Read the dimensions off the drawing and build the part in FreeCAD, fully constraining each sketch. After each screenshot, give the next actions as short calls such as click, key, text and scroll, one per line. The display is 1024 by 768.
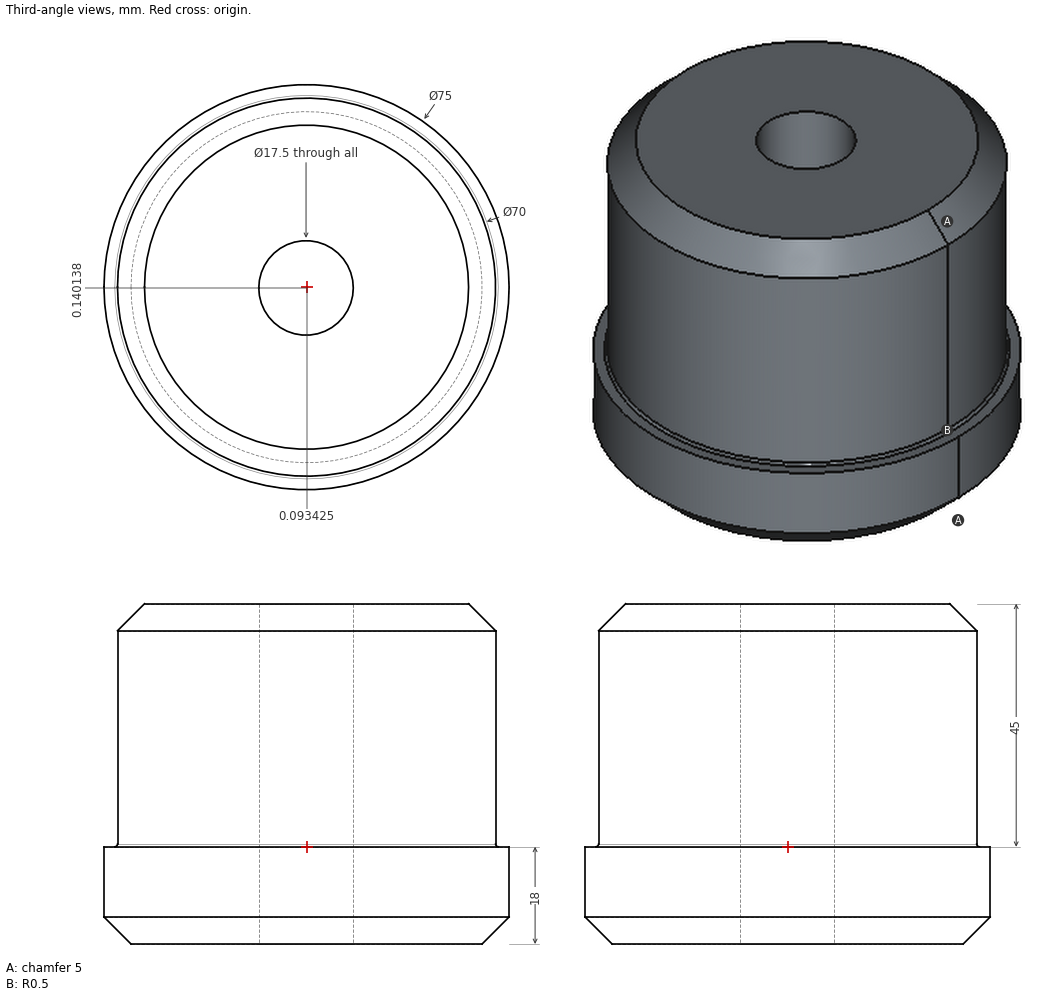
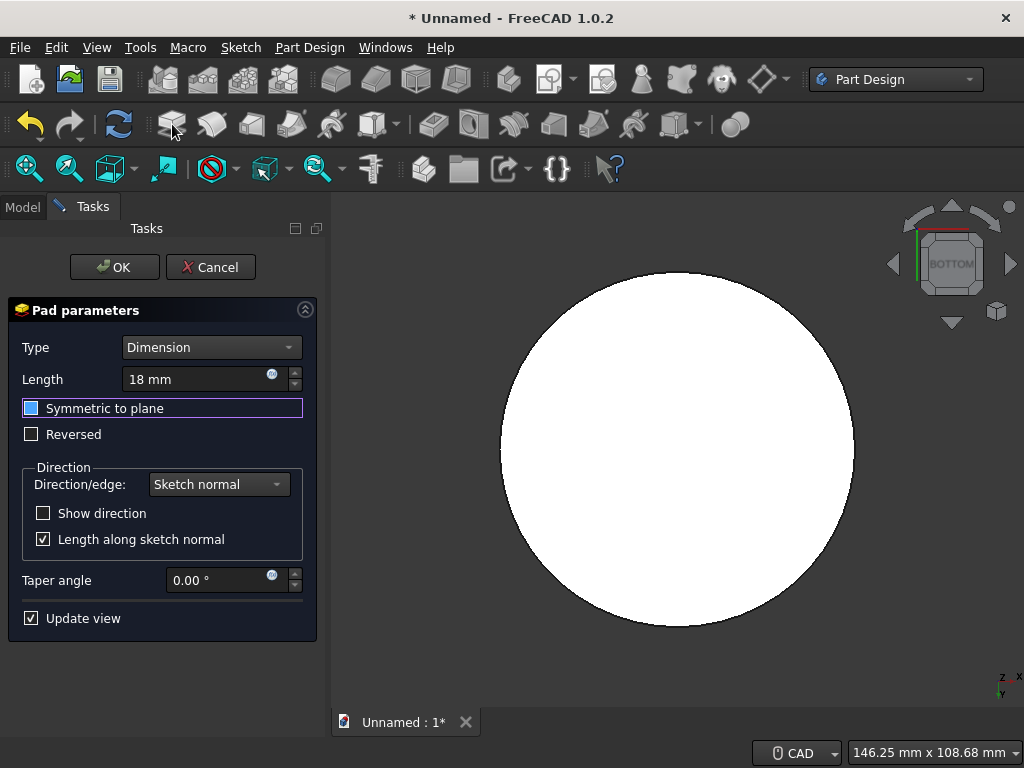
click(115, 267)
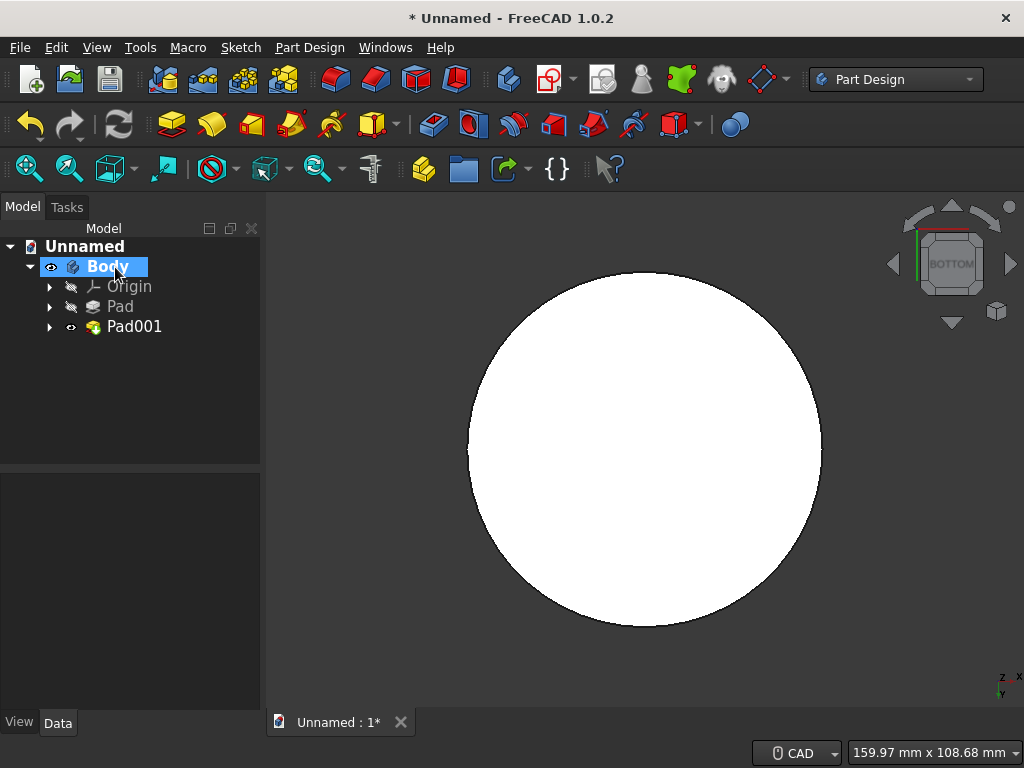
click(467, 449)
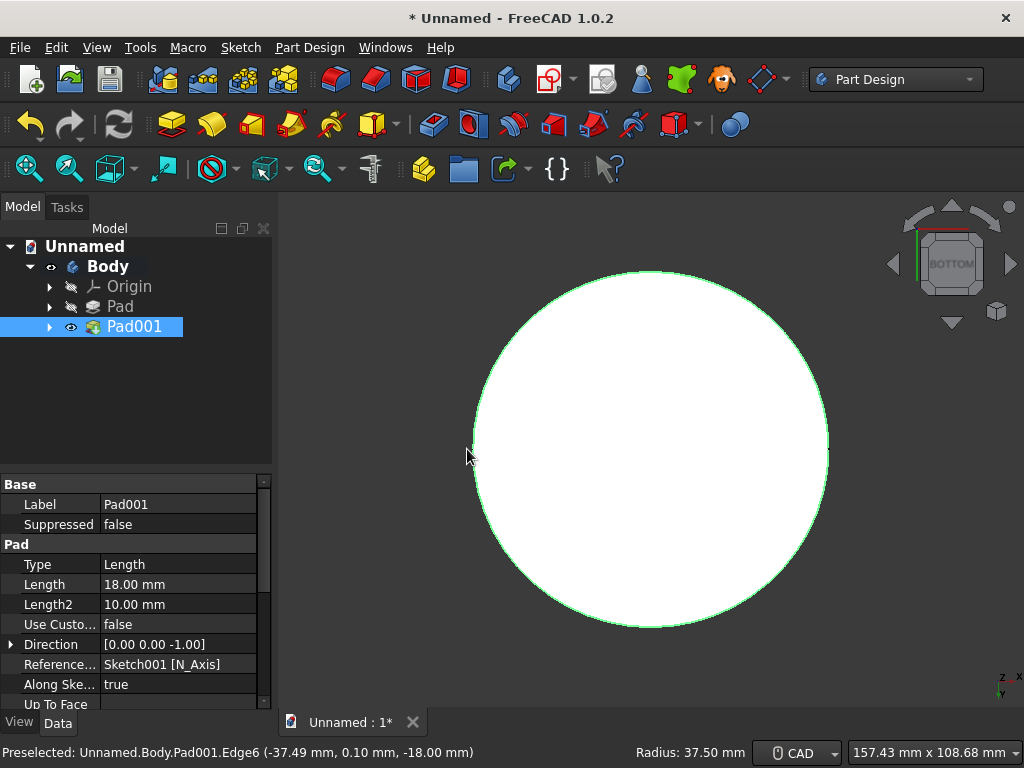
key(0)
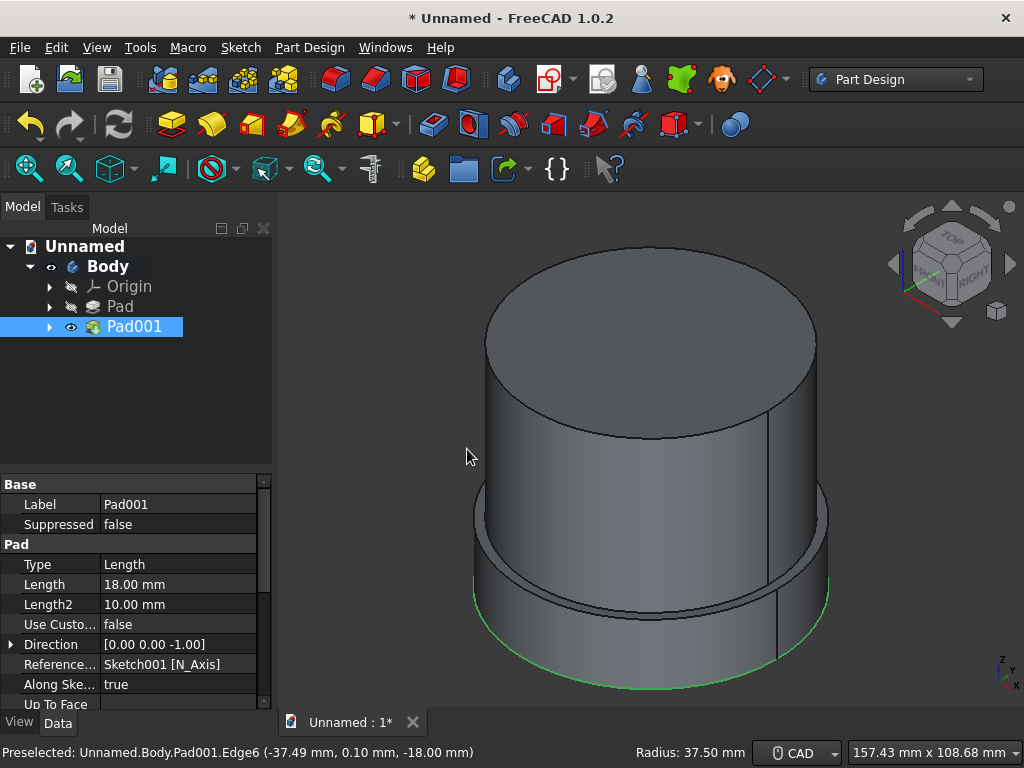
click(30, 170)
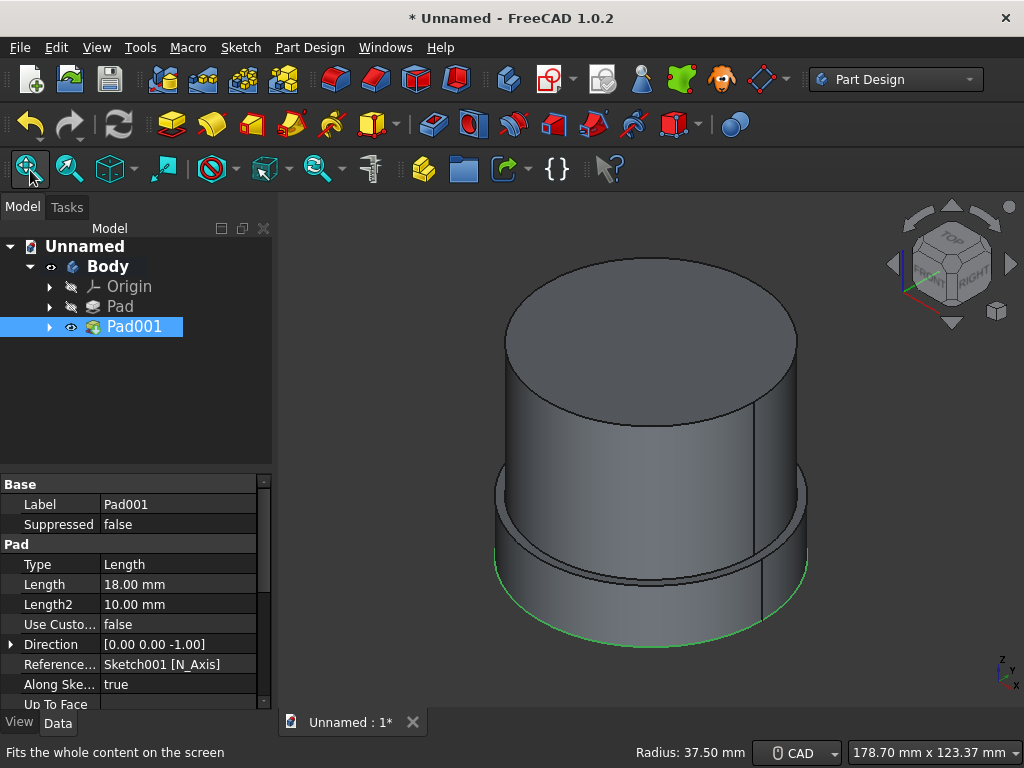
click(521, 379, ctrl)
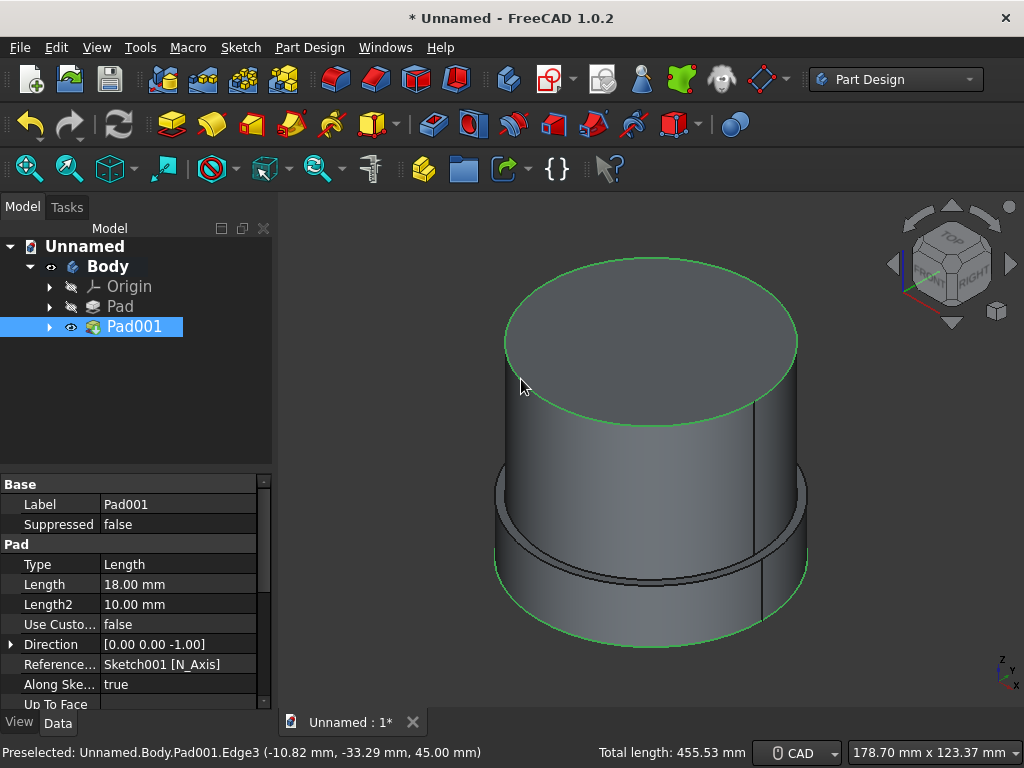
click(376, 80)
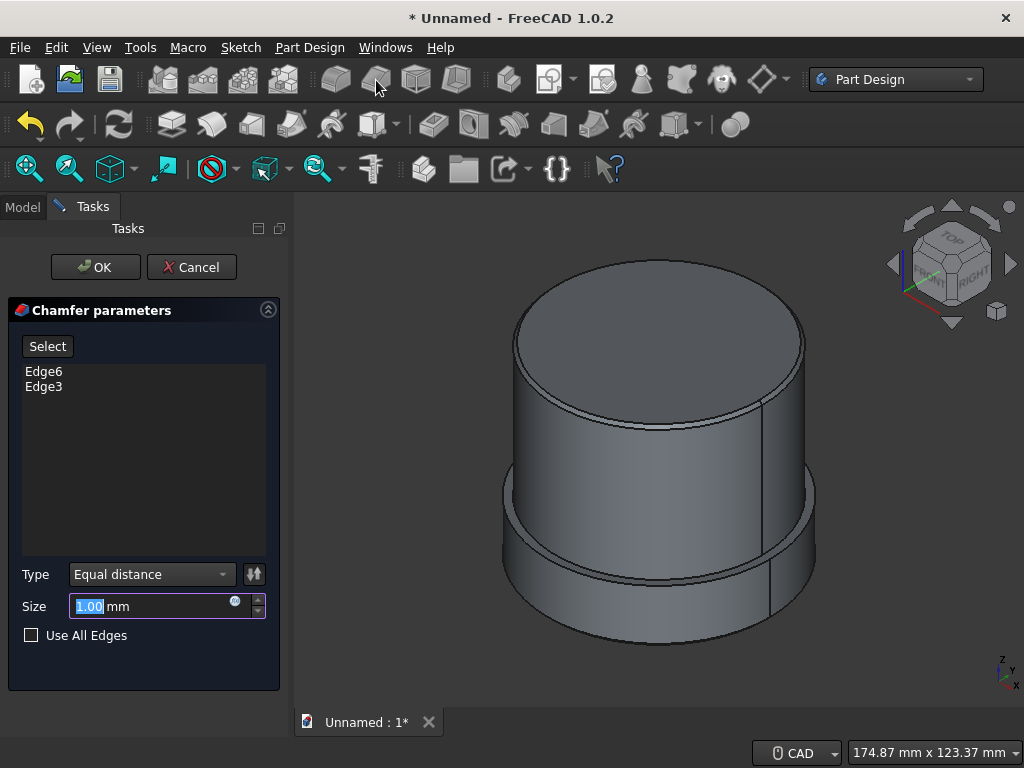
text(5)
key(Tab)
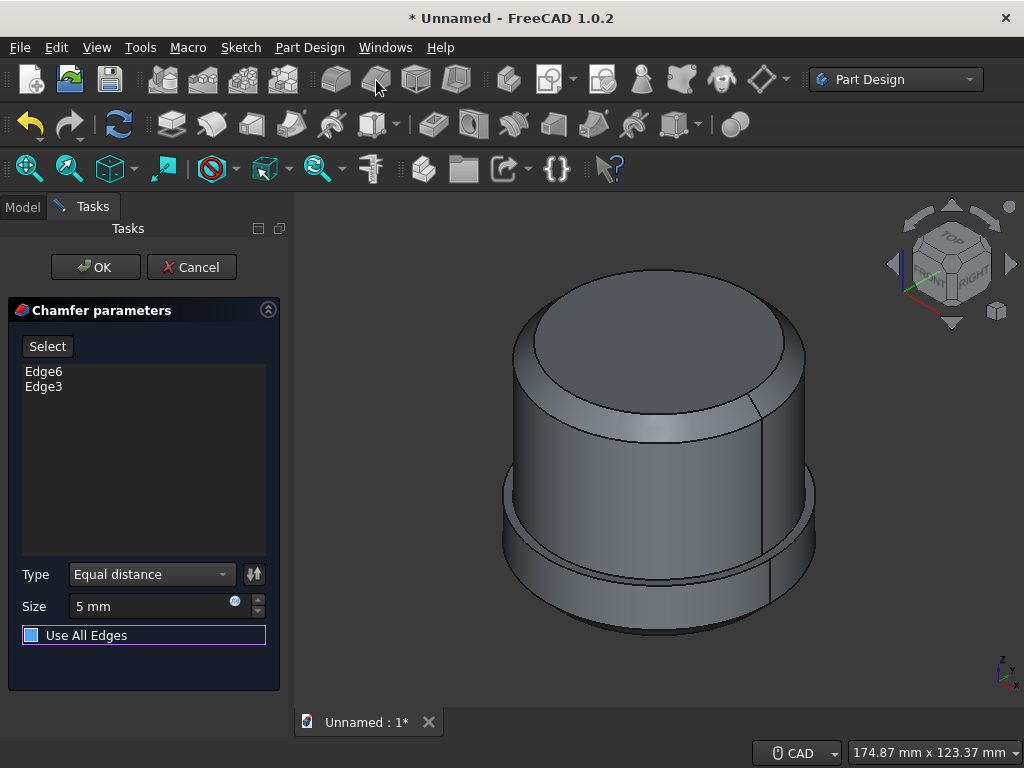
click(96, 267)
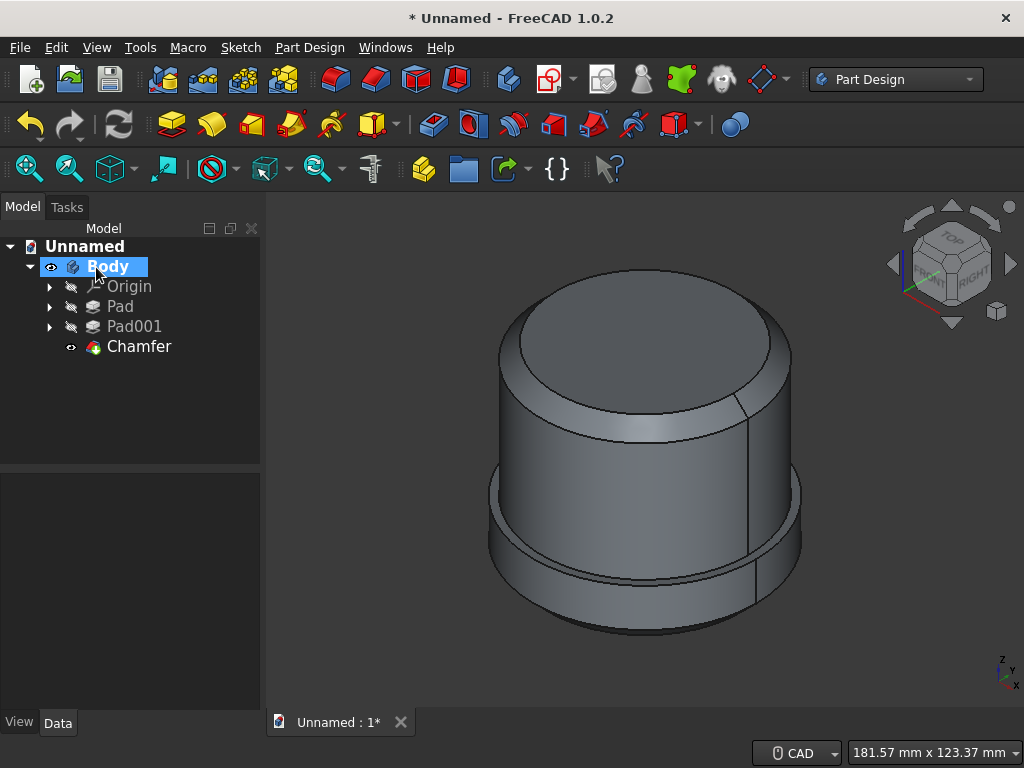
click(645, 341)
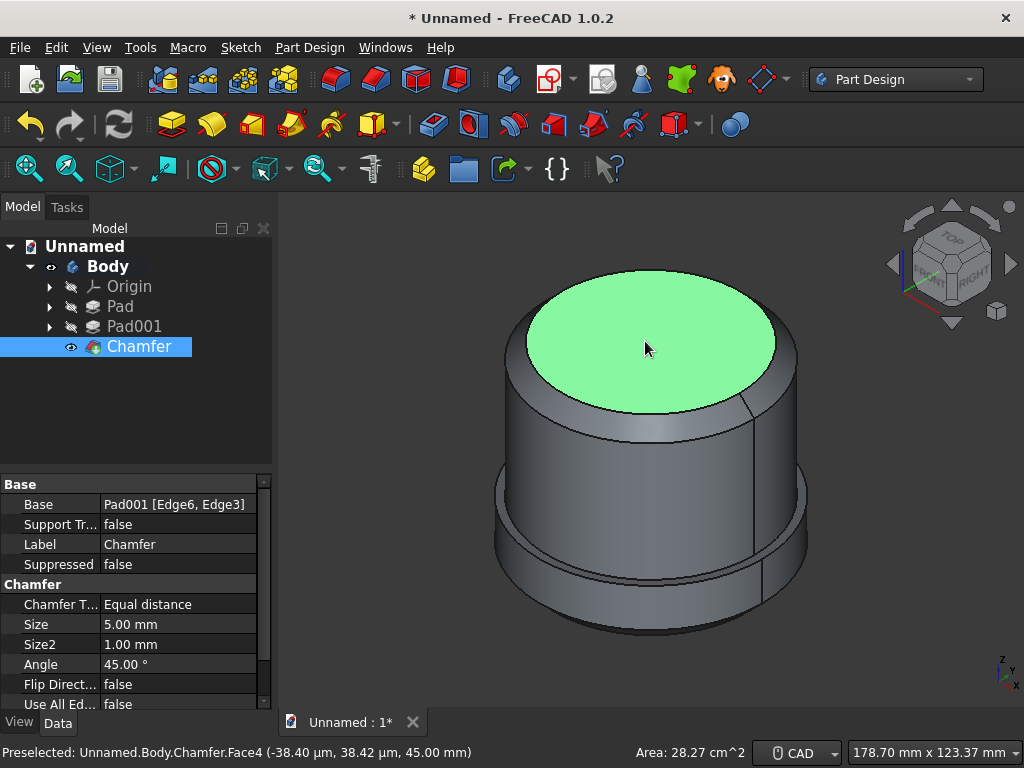
click(550, 80)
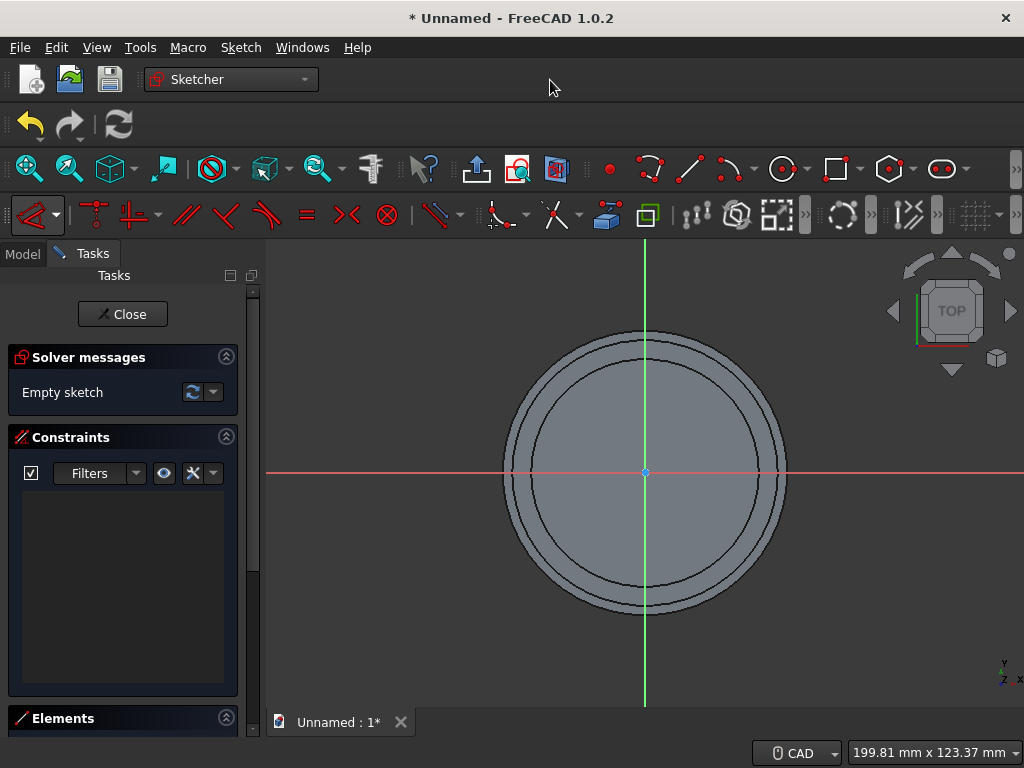
scroll(667, 474, up, 7)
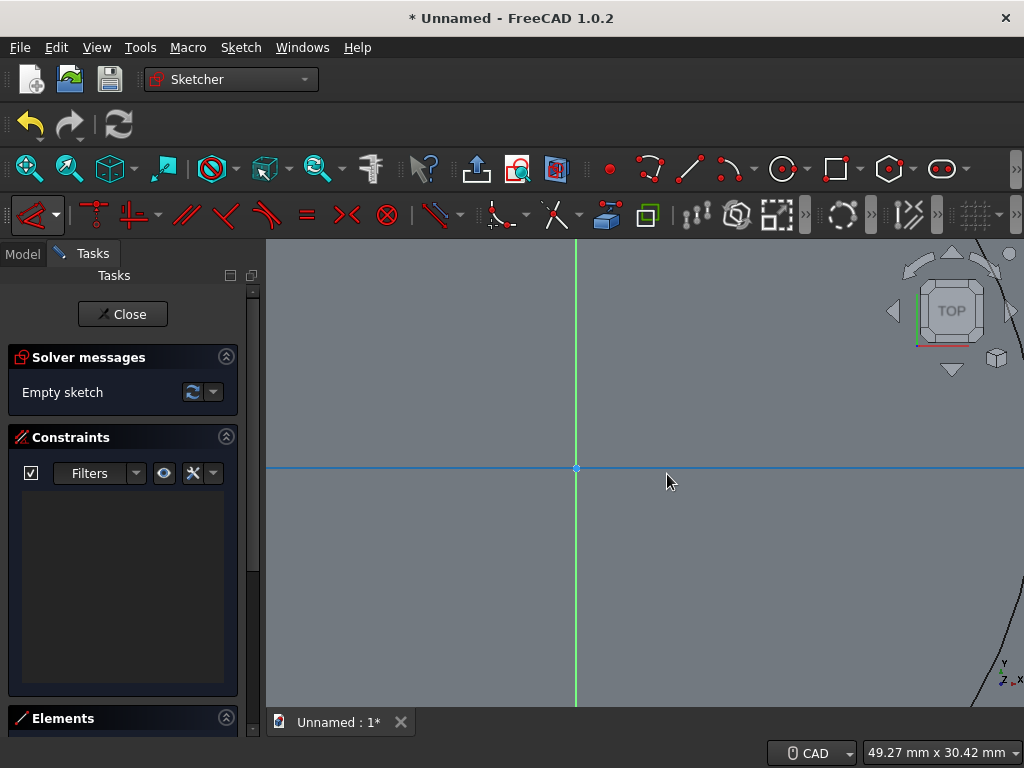
click(784, 170)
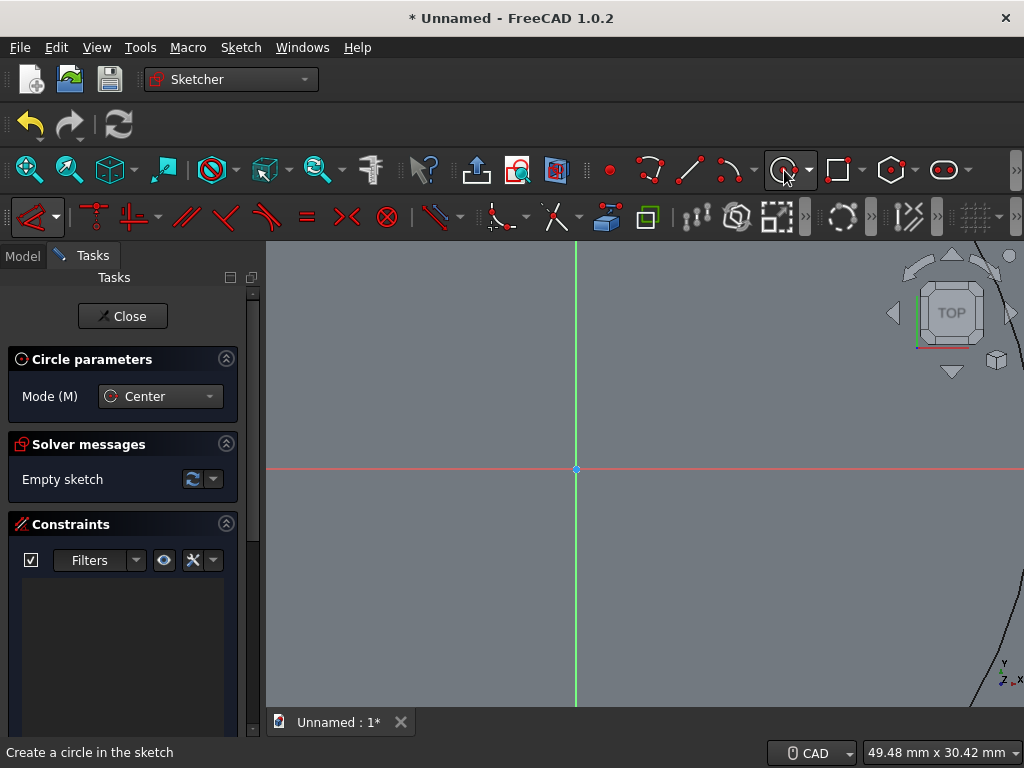
scroll(575, 472, up, 13)